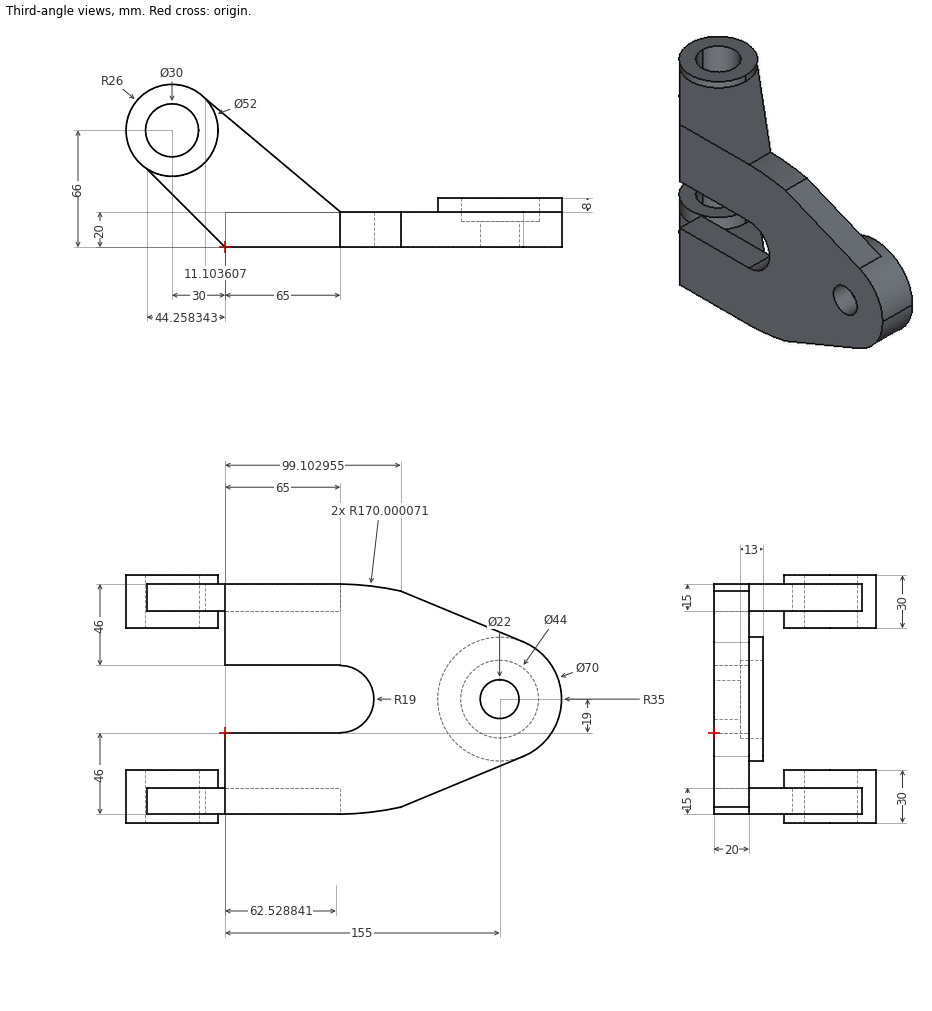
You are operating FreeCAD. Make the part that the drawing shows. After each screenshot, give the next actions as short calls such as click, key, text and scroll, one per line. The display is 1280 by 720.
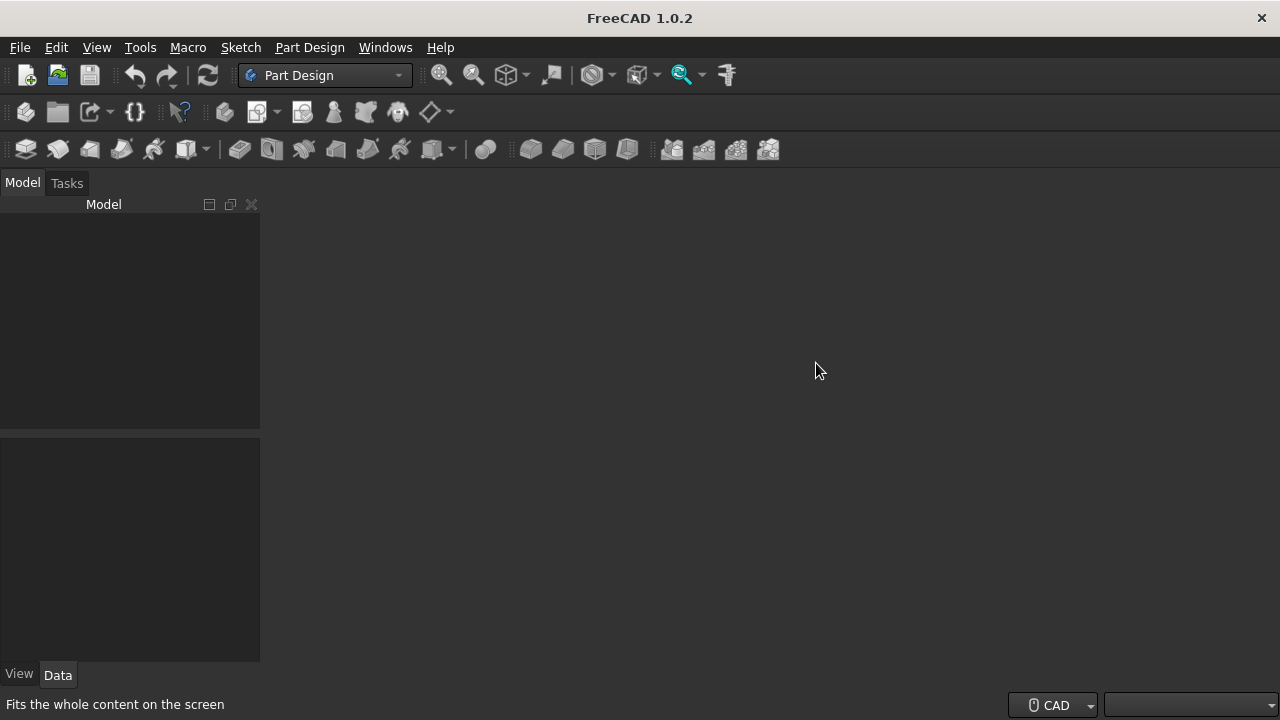
key(ctrl+n)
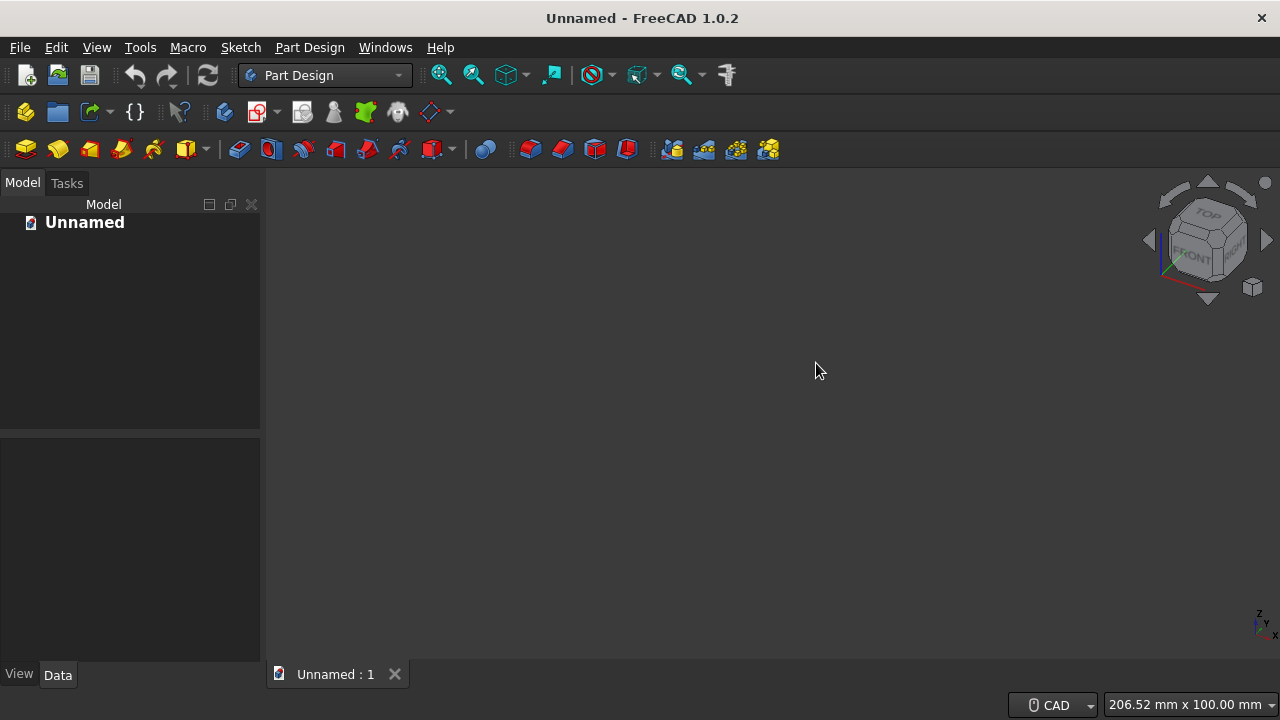
click(258, 112)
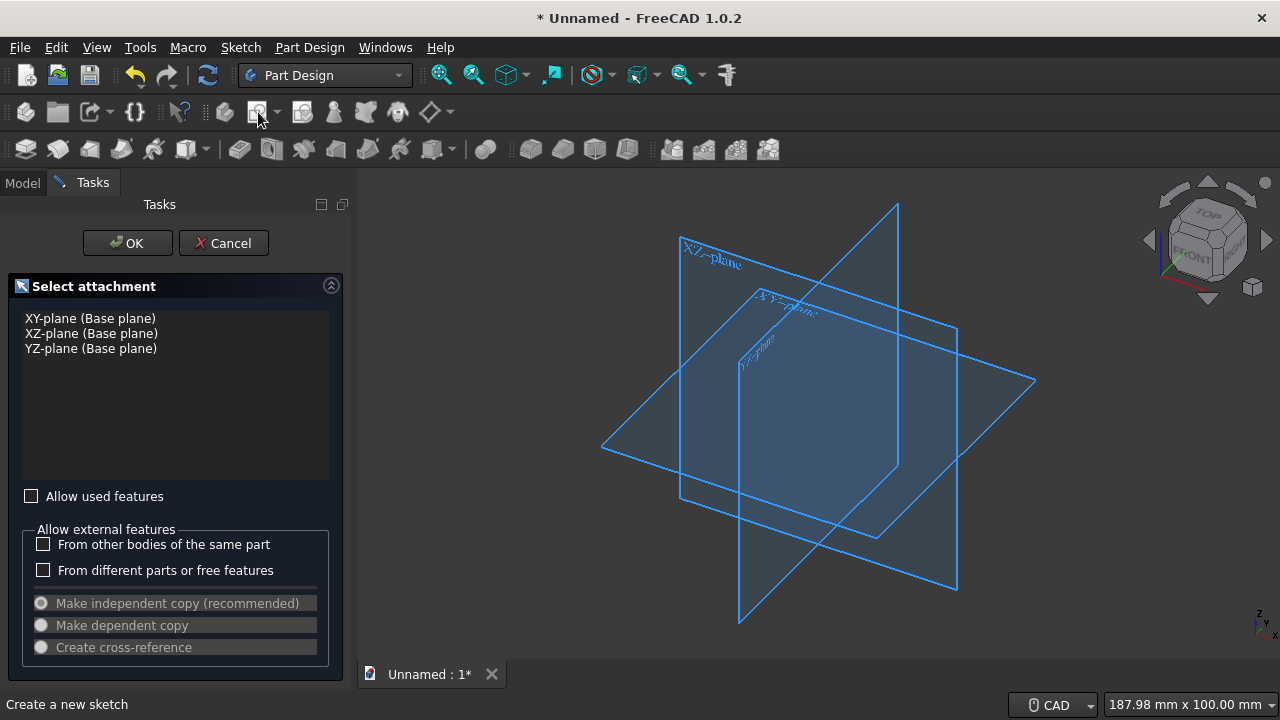
click(82, 334)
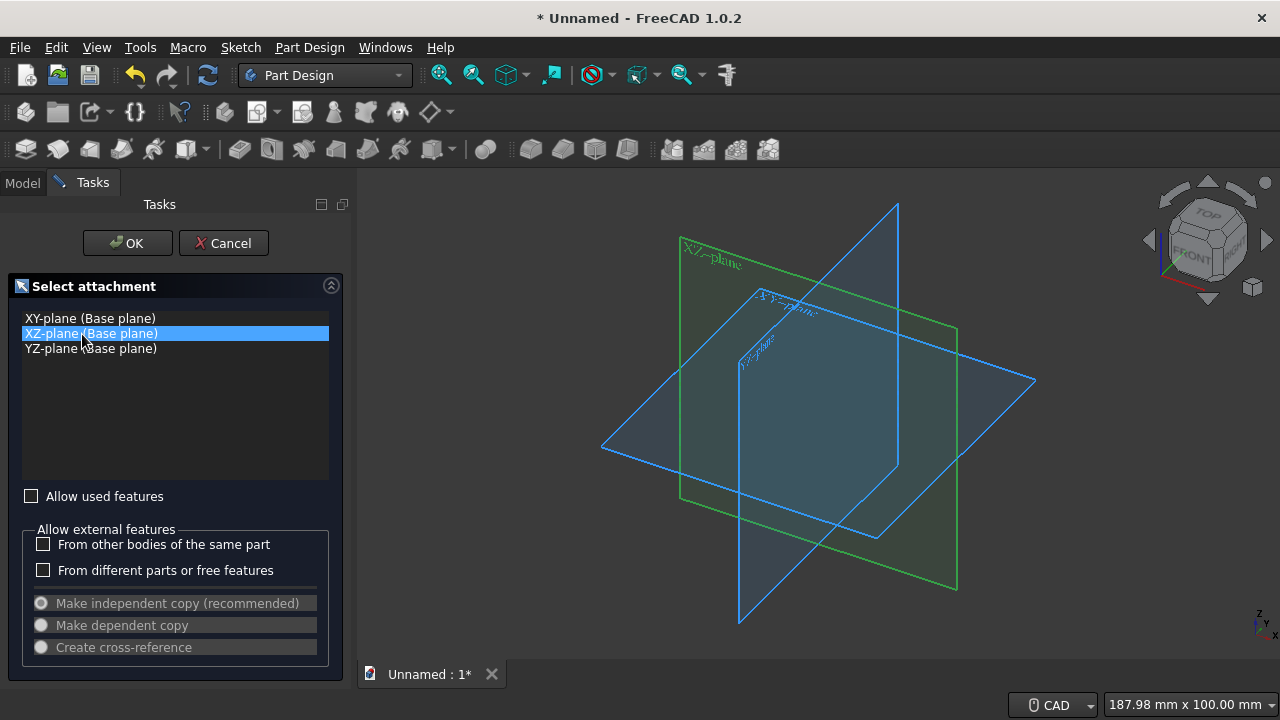
click(128, 243)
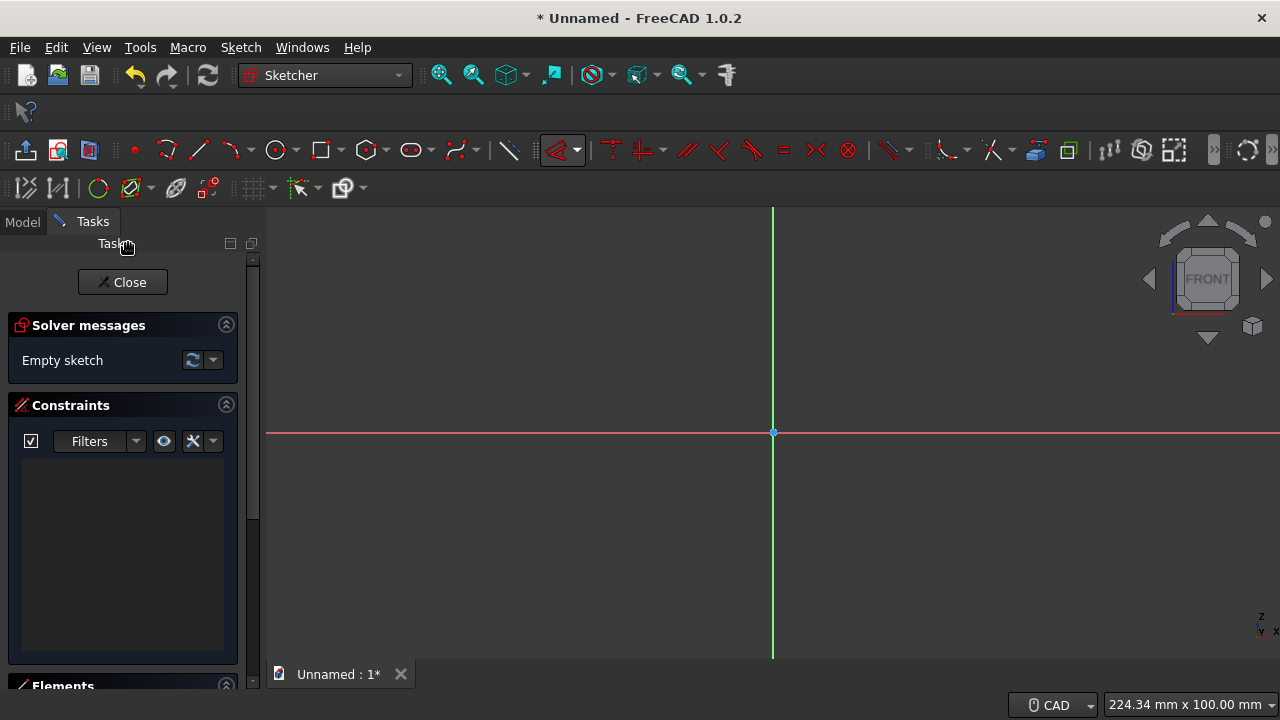
scroll(298, 503, down, 4)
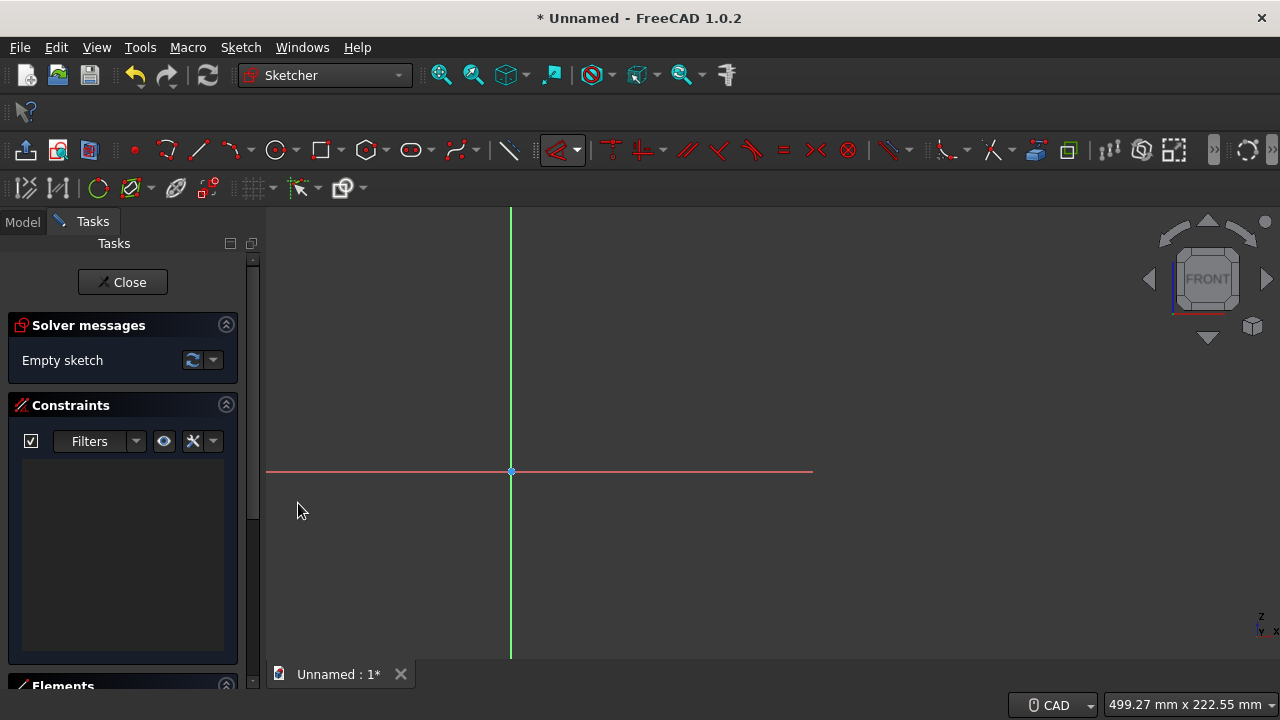
click(168, 150)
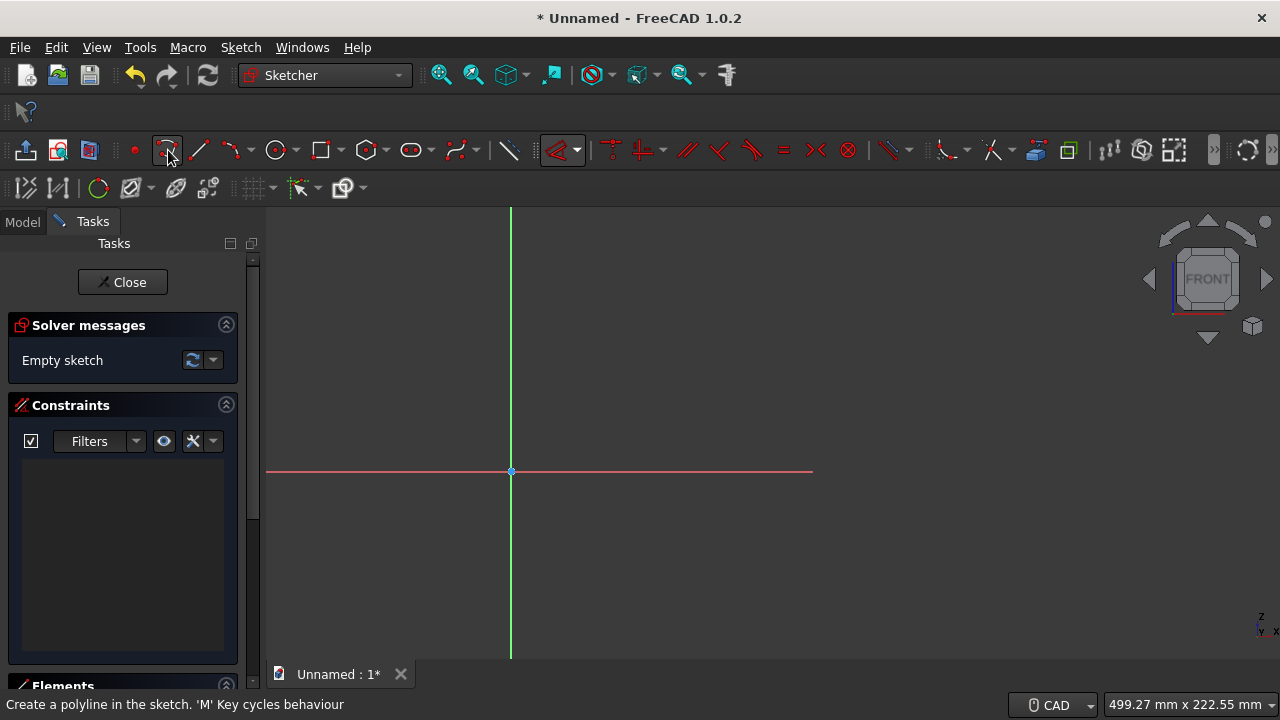
click(643, 395)
click(511, 395)
click(520, 301)
click(643, 301)
right_click(643, 301)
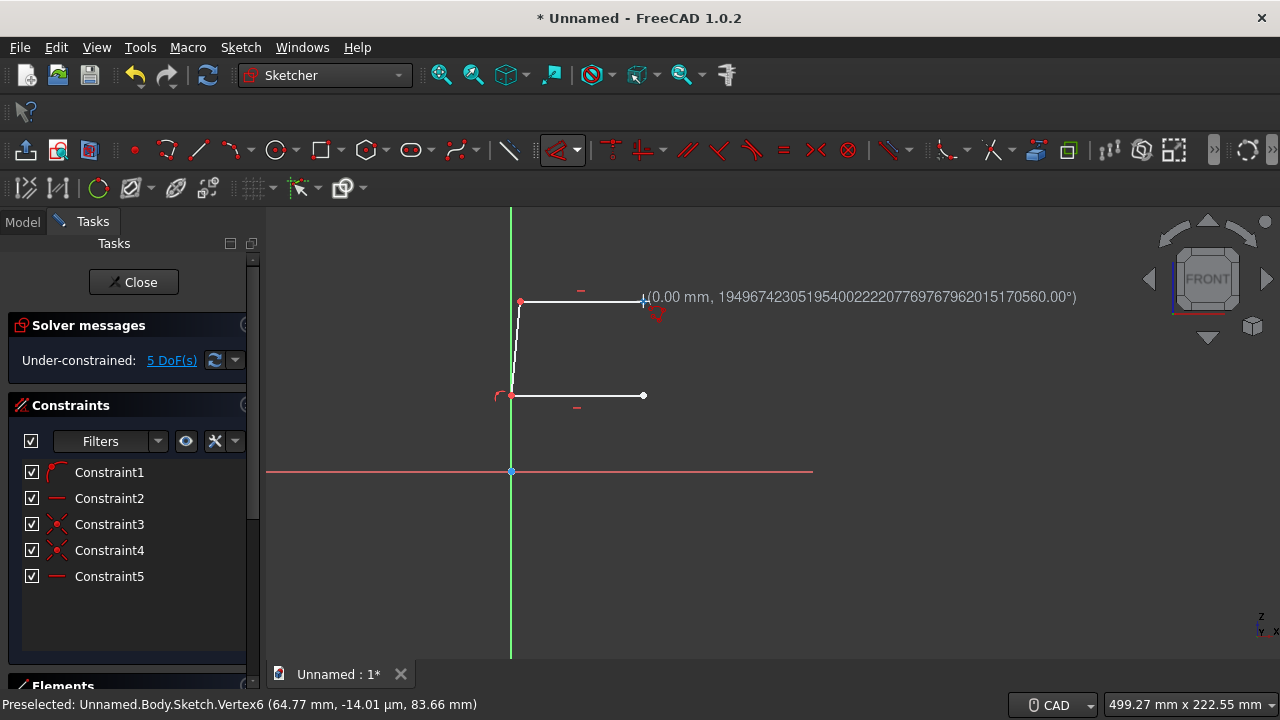
key(g)
key(l)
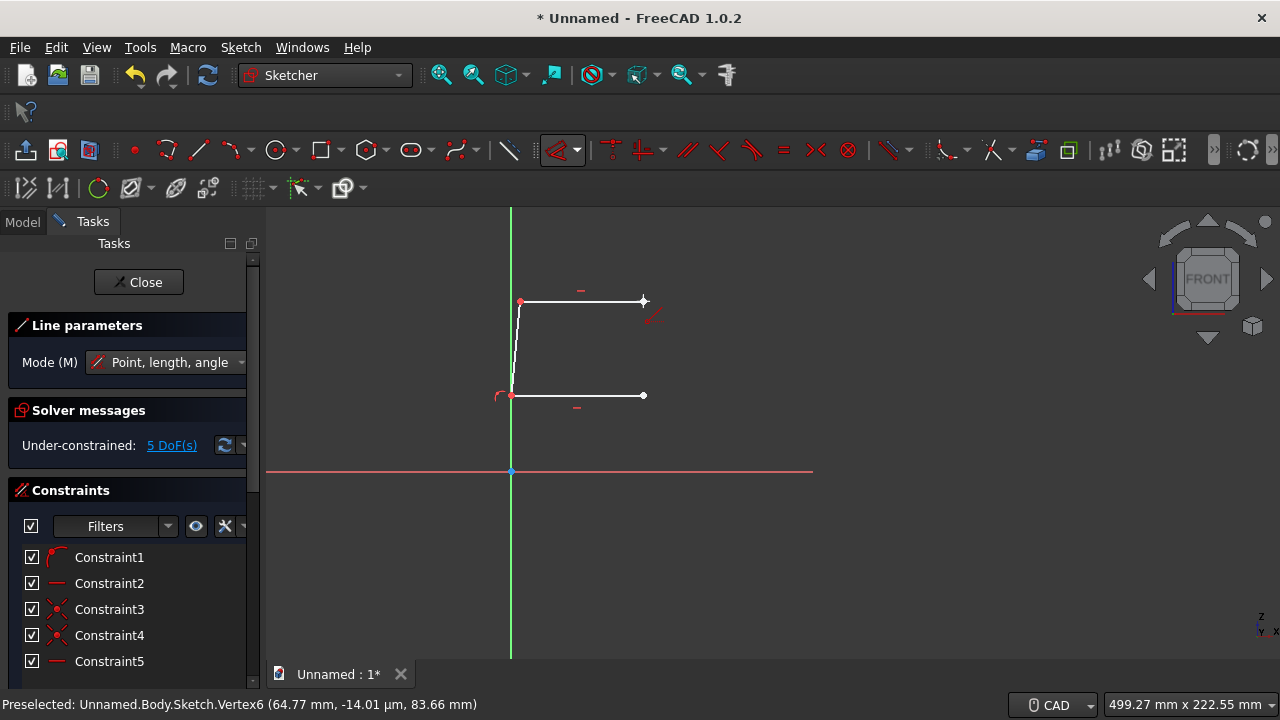
click(713, 309)
click(853, 368)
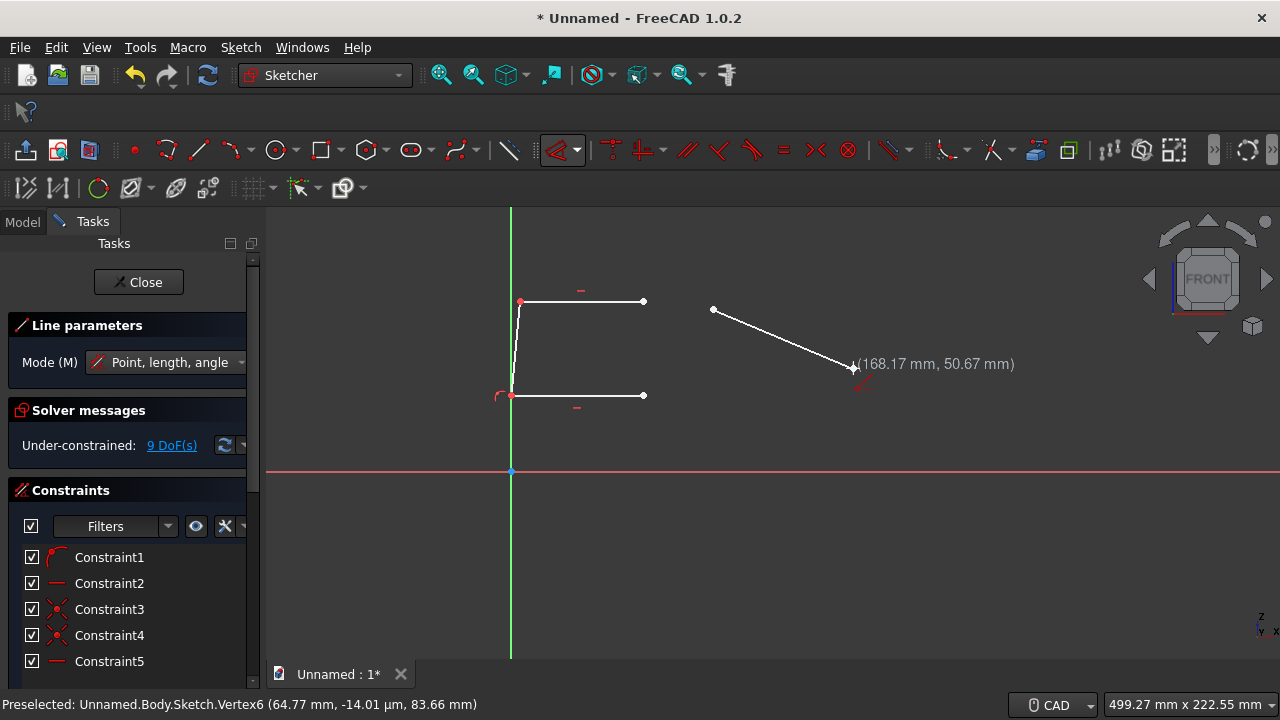
click(853, 499)
click(713, 557)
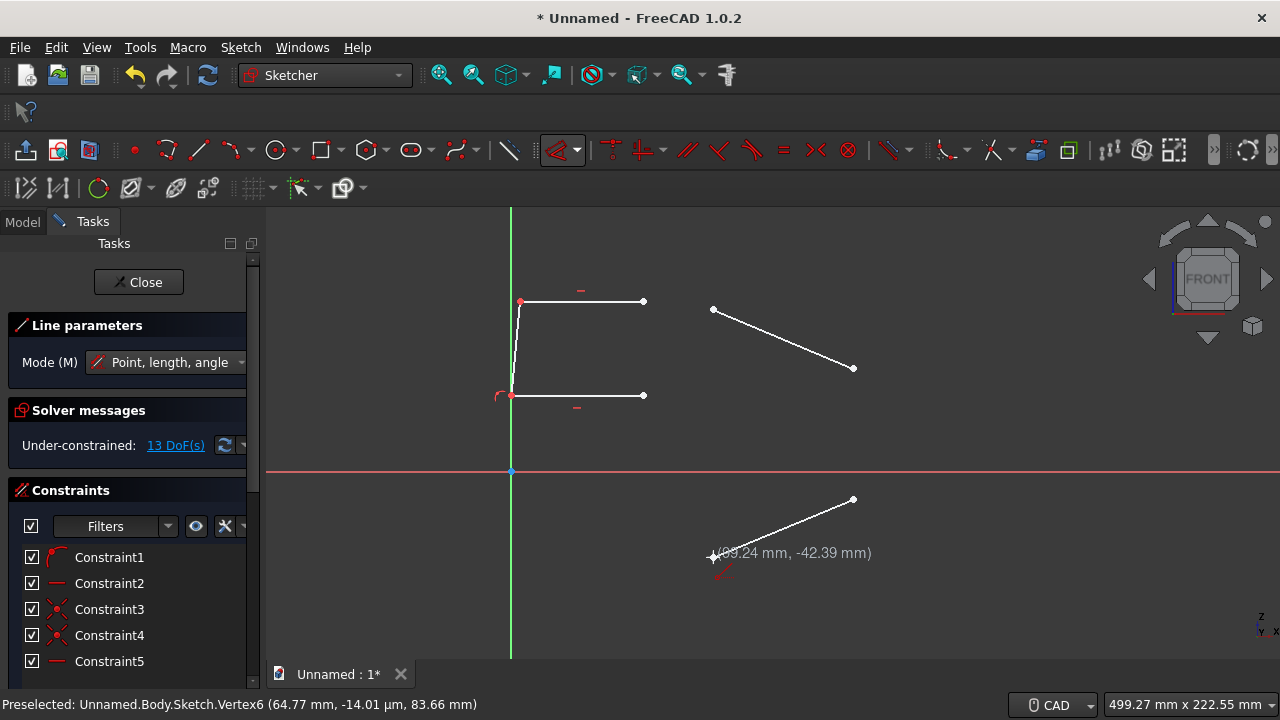
click(168, 150)